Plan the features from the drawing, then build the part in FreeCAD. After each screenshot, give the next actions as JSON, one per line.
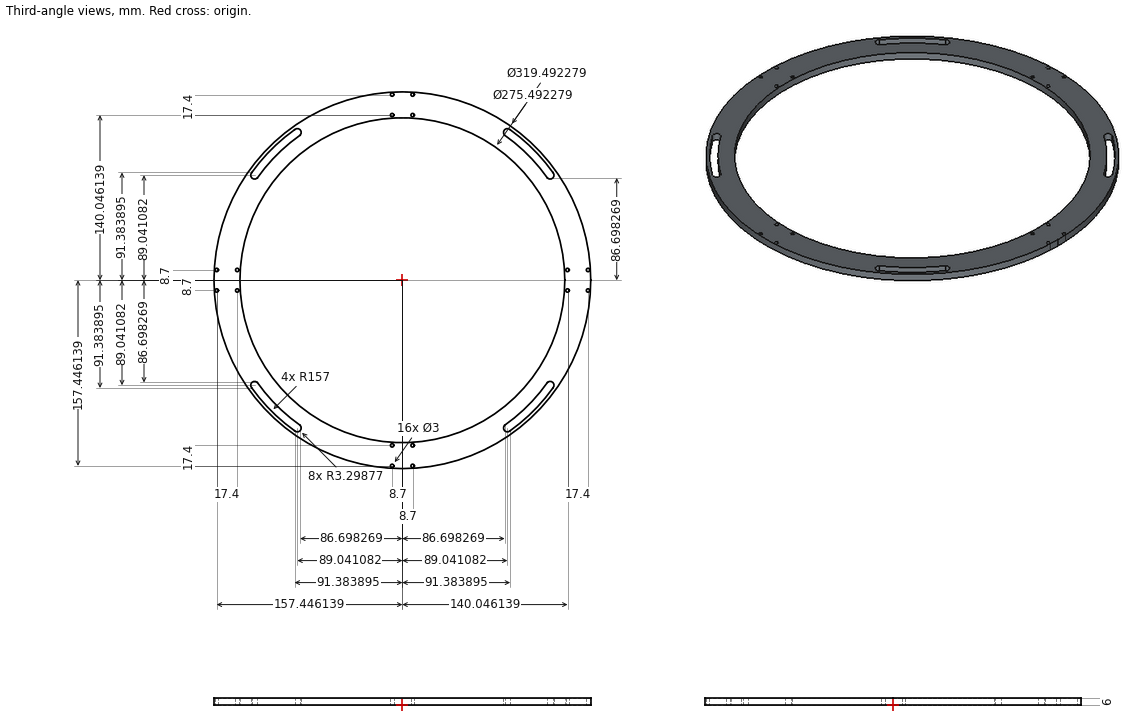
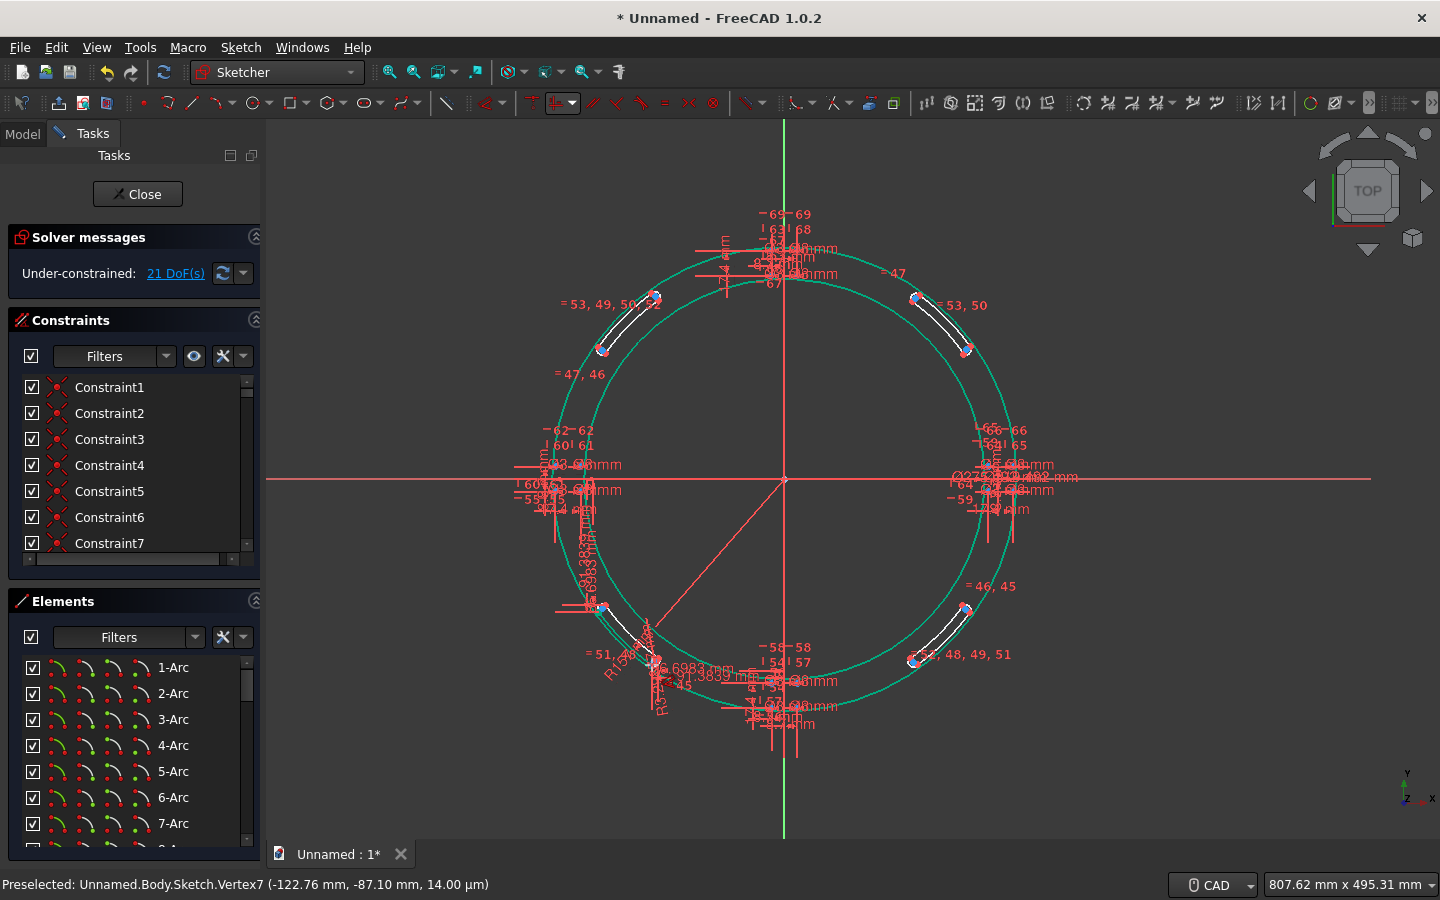
{"action": "scroll", "coordinate": [970, 613], "scroll_direction": "up", "scroll_amount": 5}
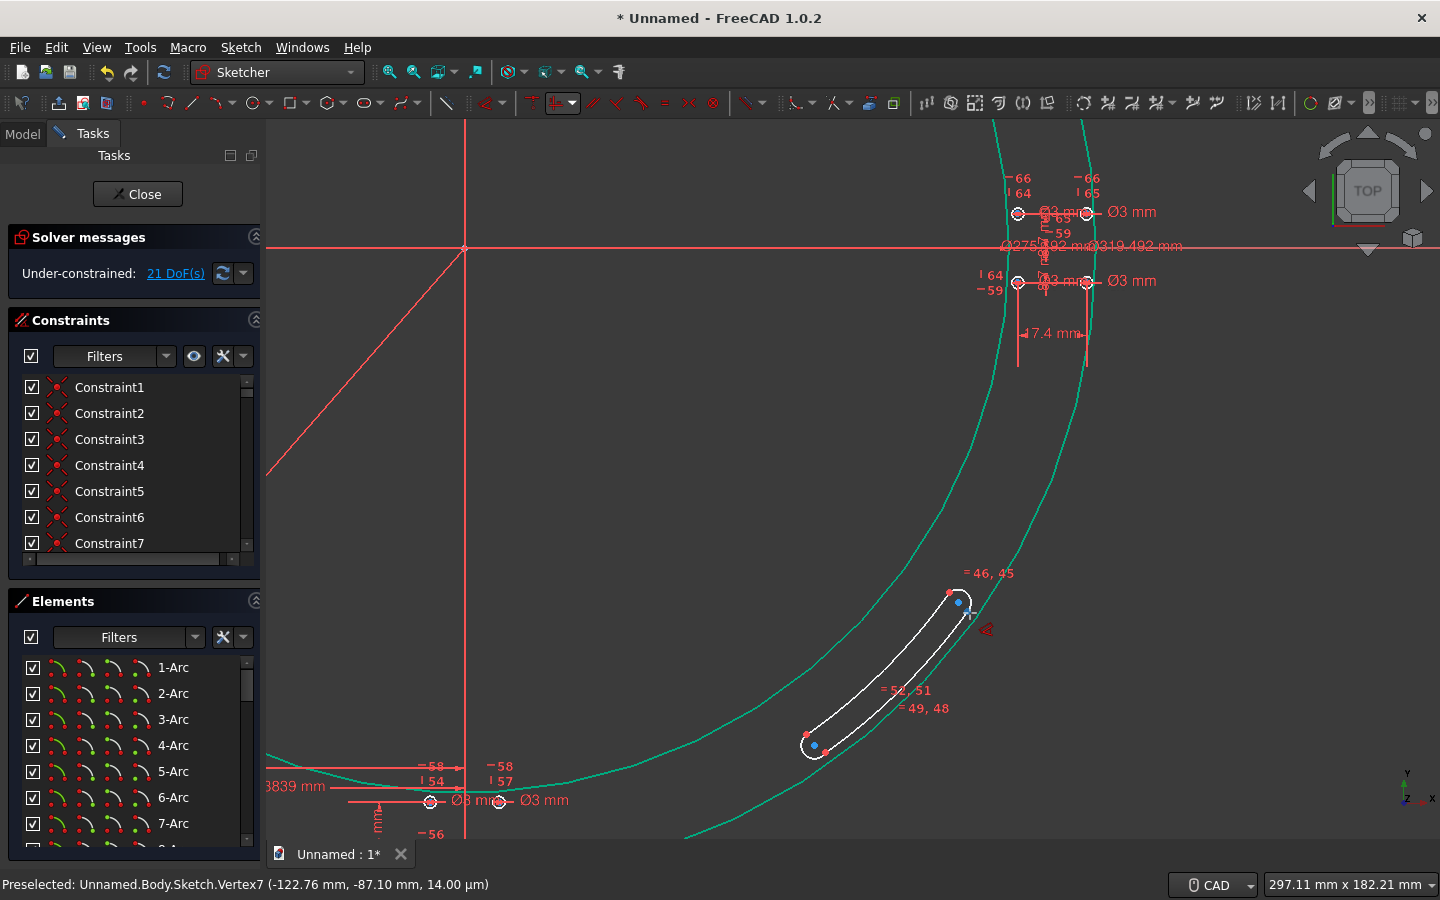
{"action": "left_click", "coordinate": [968, 611]}
{"action": "left_click", "coordinate": [1002, 430]}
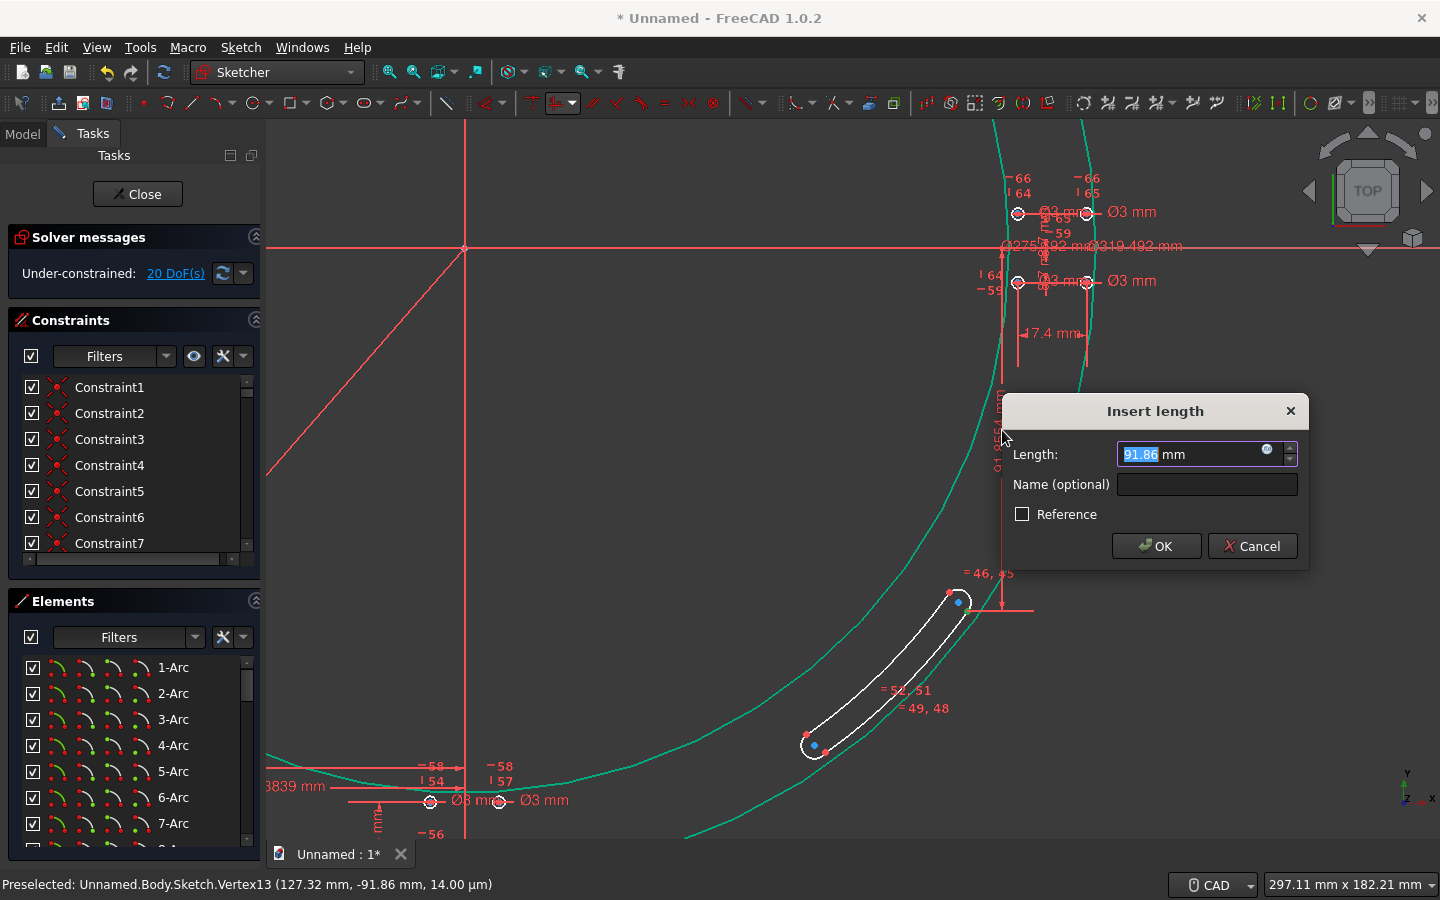
{"action": "type", "text": "91.383895"}
{"action": "key", "text": "Return"}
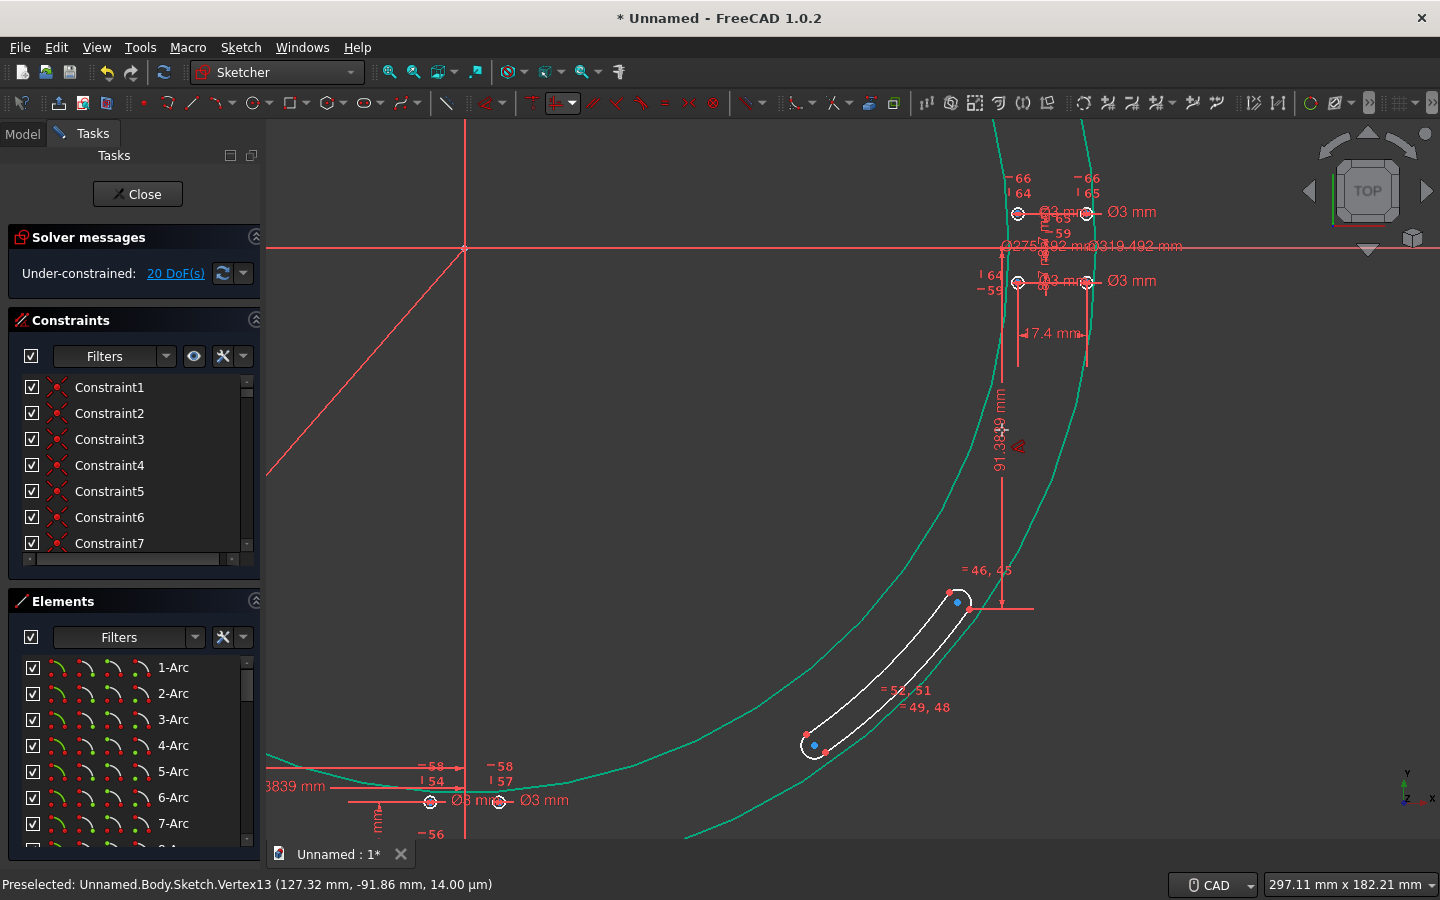
{"action": "left_click", "coordinate": [826, 753]}
{"action": "left_click", "coordinate": [645, 787]}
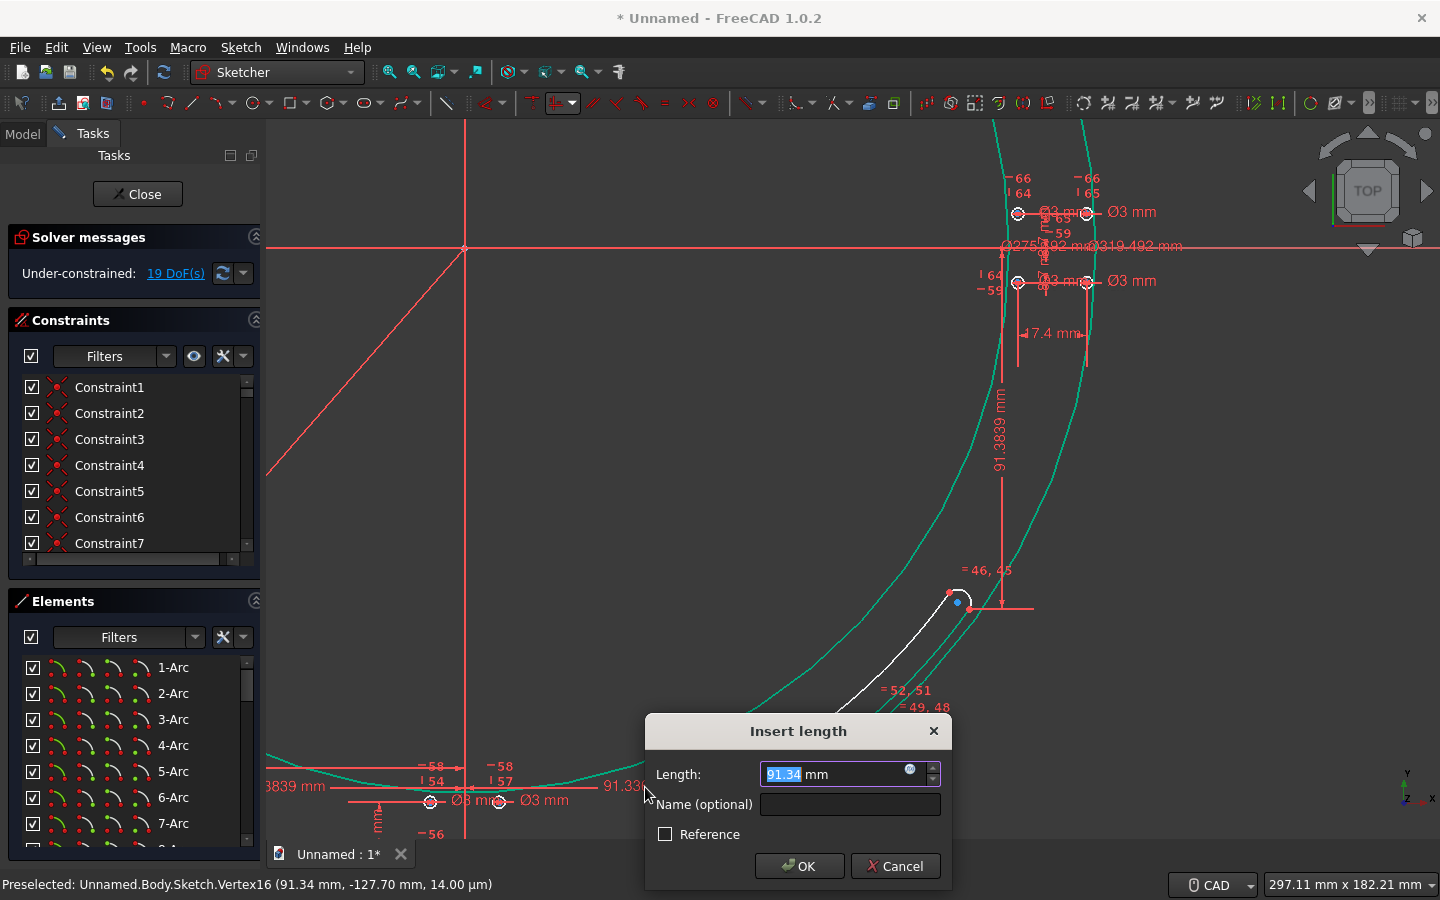
{"action": "type", "text": "91.383895"}
{"action": "key", "text": "Return"}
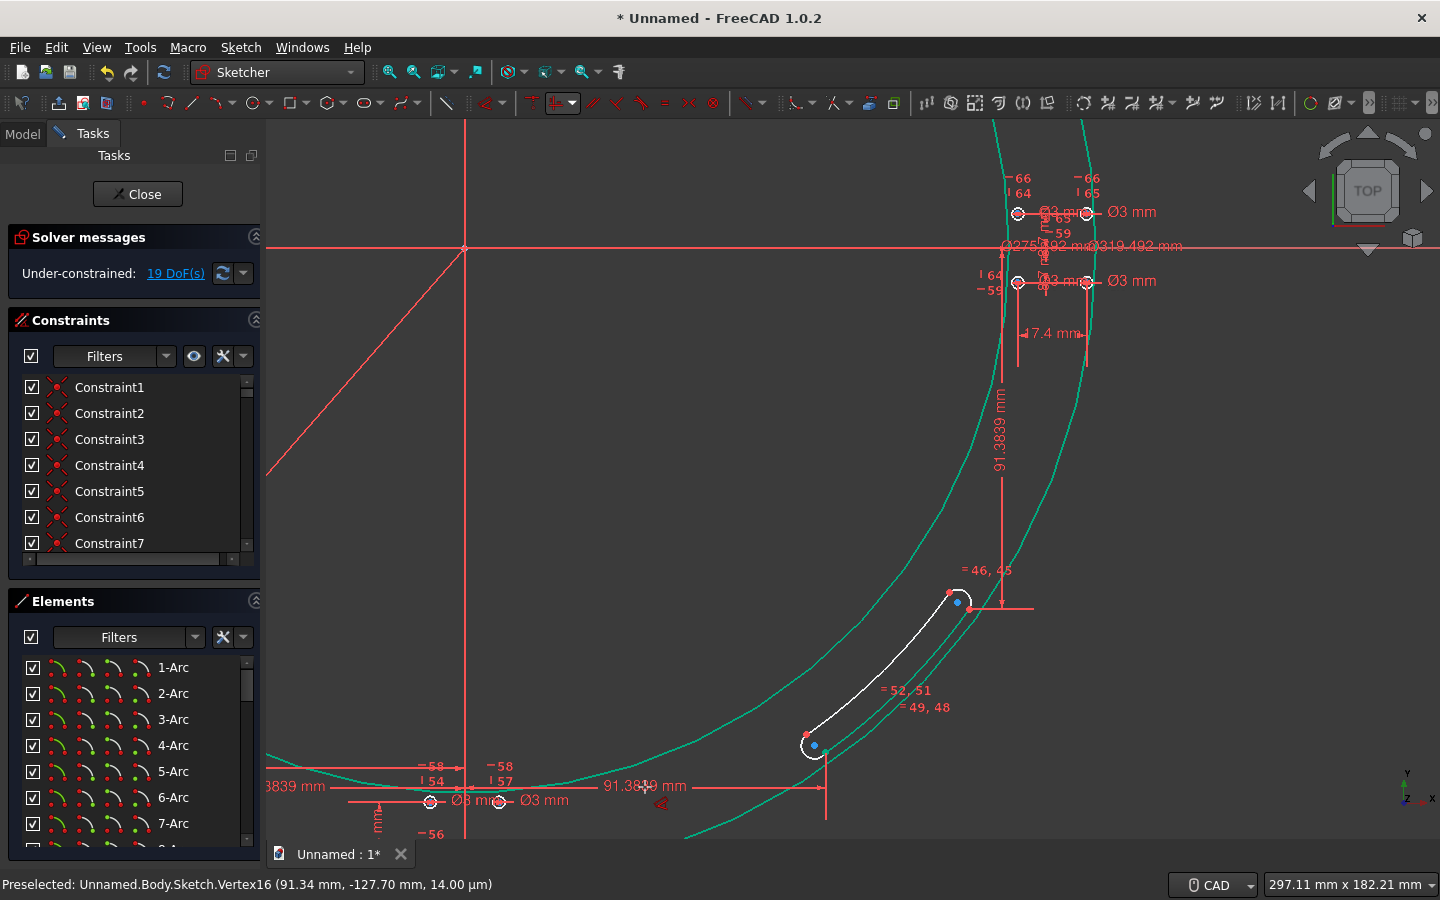
{"action": "left_click", "coordinate": [807, 735]}
{"action": "left_click", "coordinate": [557, 769]}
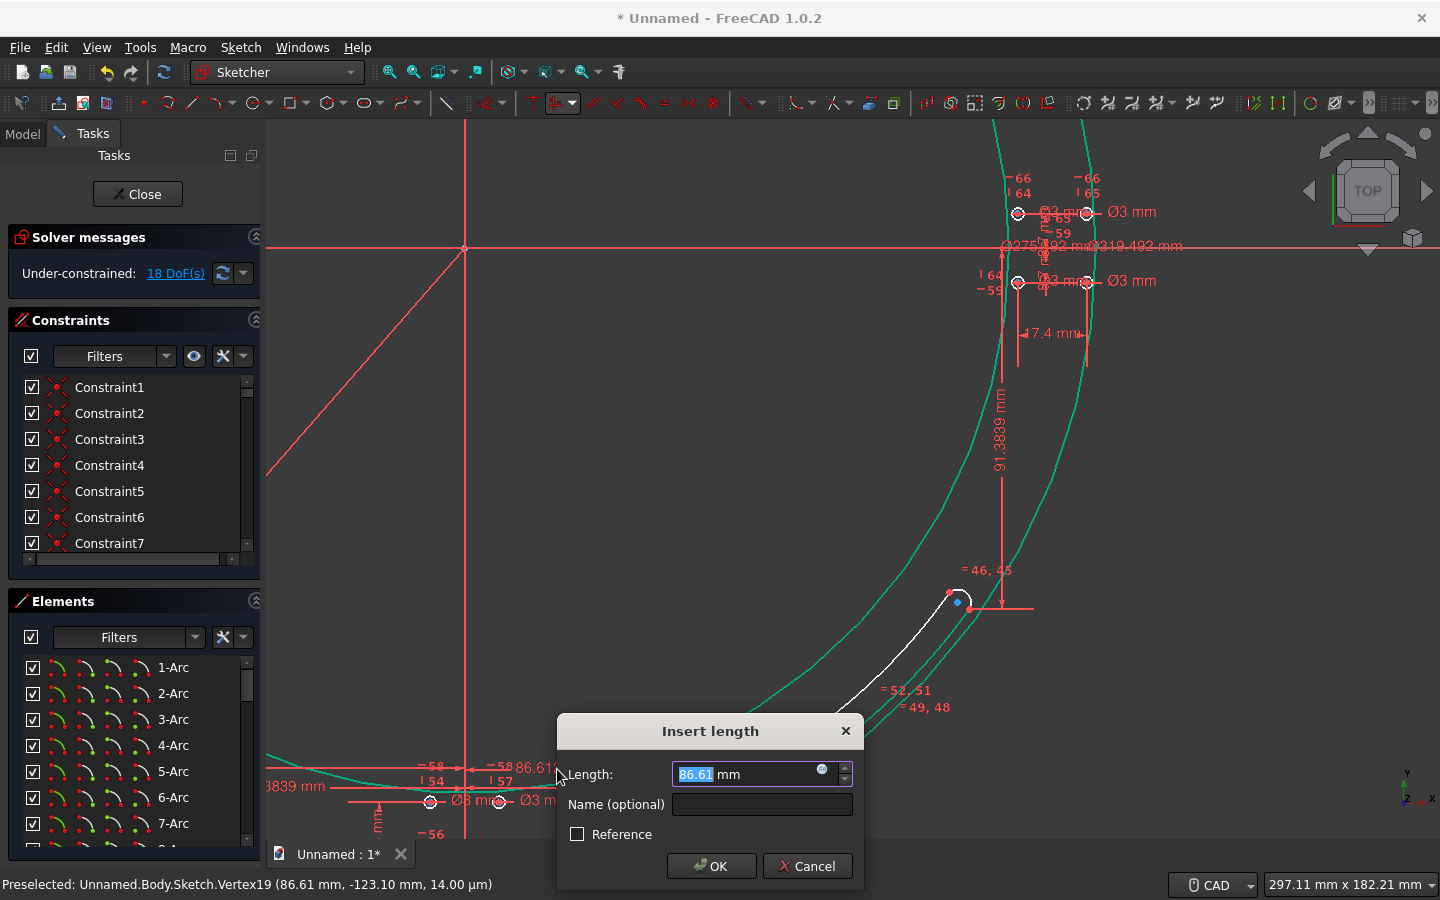
{"action": "type", "text": "86.698269"}
{"action": "key", "text": "Return"}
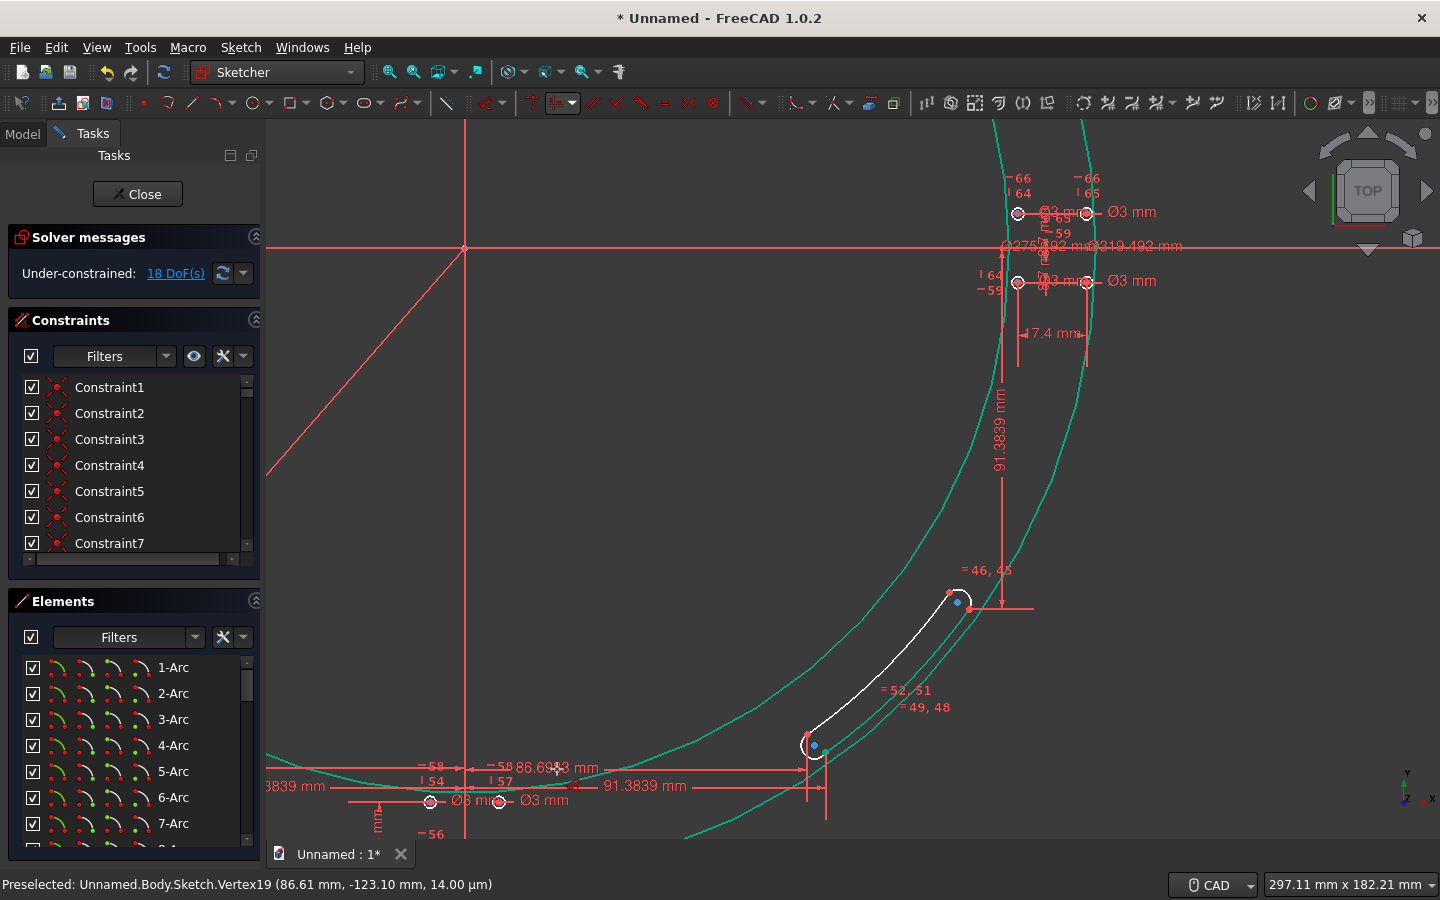
{"action": "scroll", "coordinate": [971, 613], "scroll_direction": "down", "scroll_amount": 5}